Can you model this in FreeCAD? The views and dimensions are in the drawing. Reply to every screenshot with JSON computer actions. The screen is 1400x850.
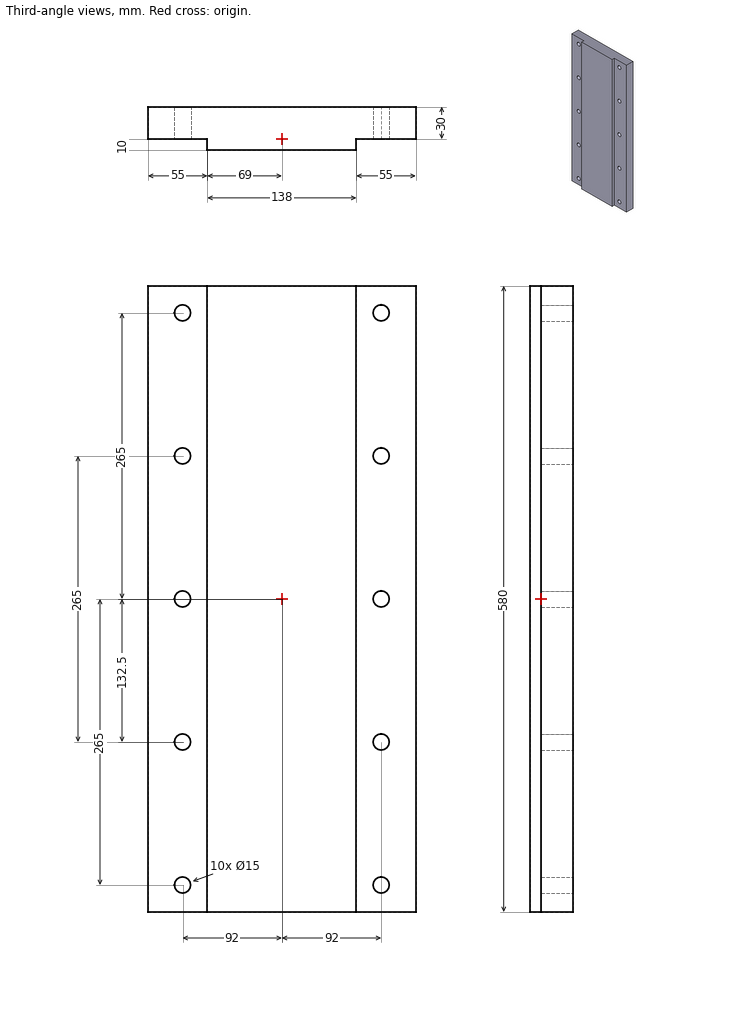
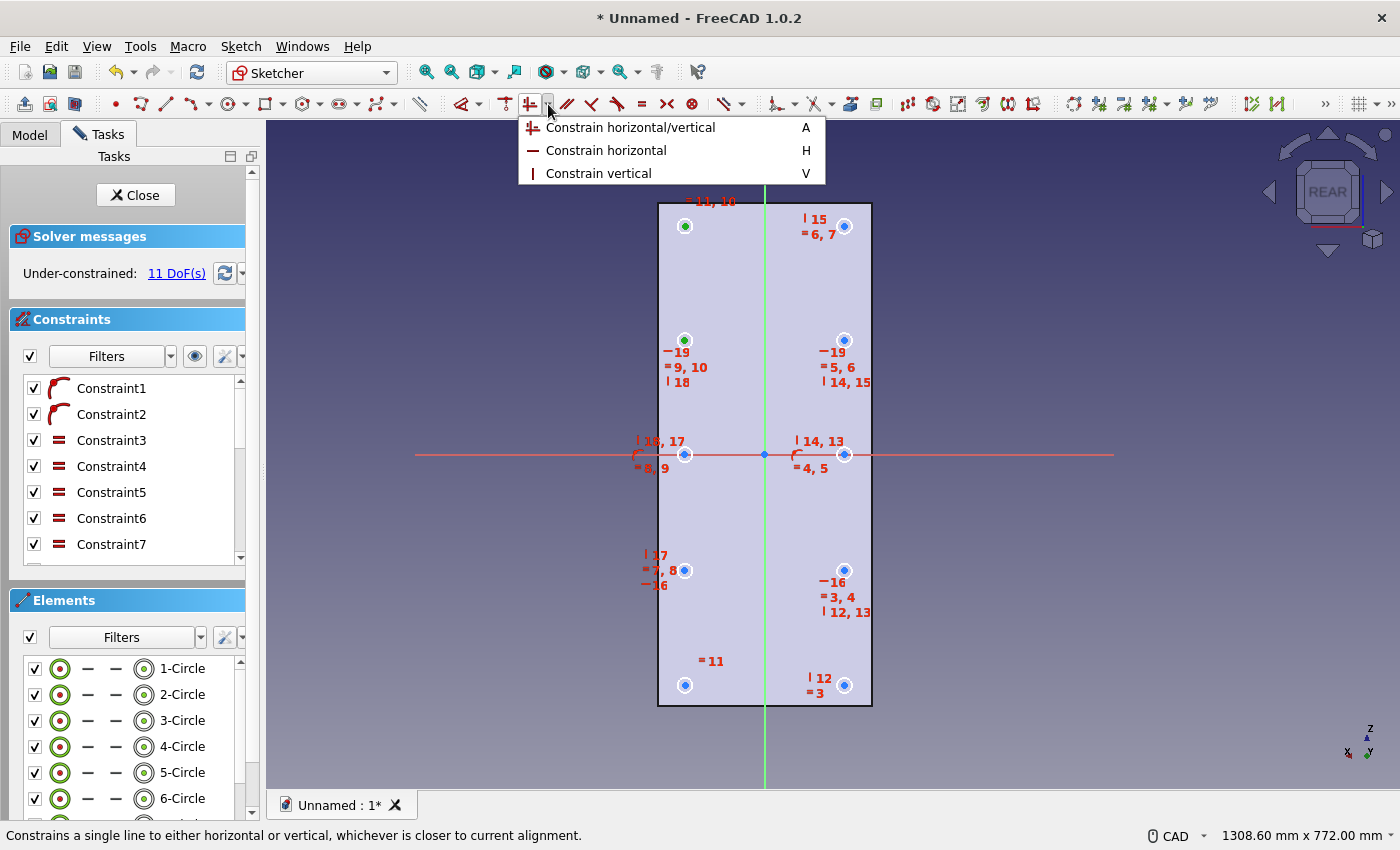
{"action": "left_click", "coordinate": [672, 174]}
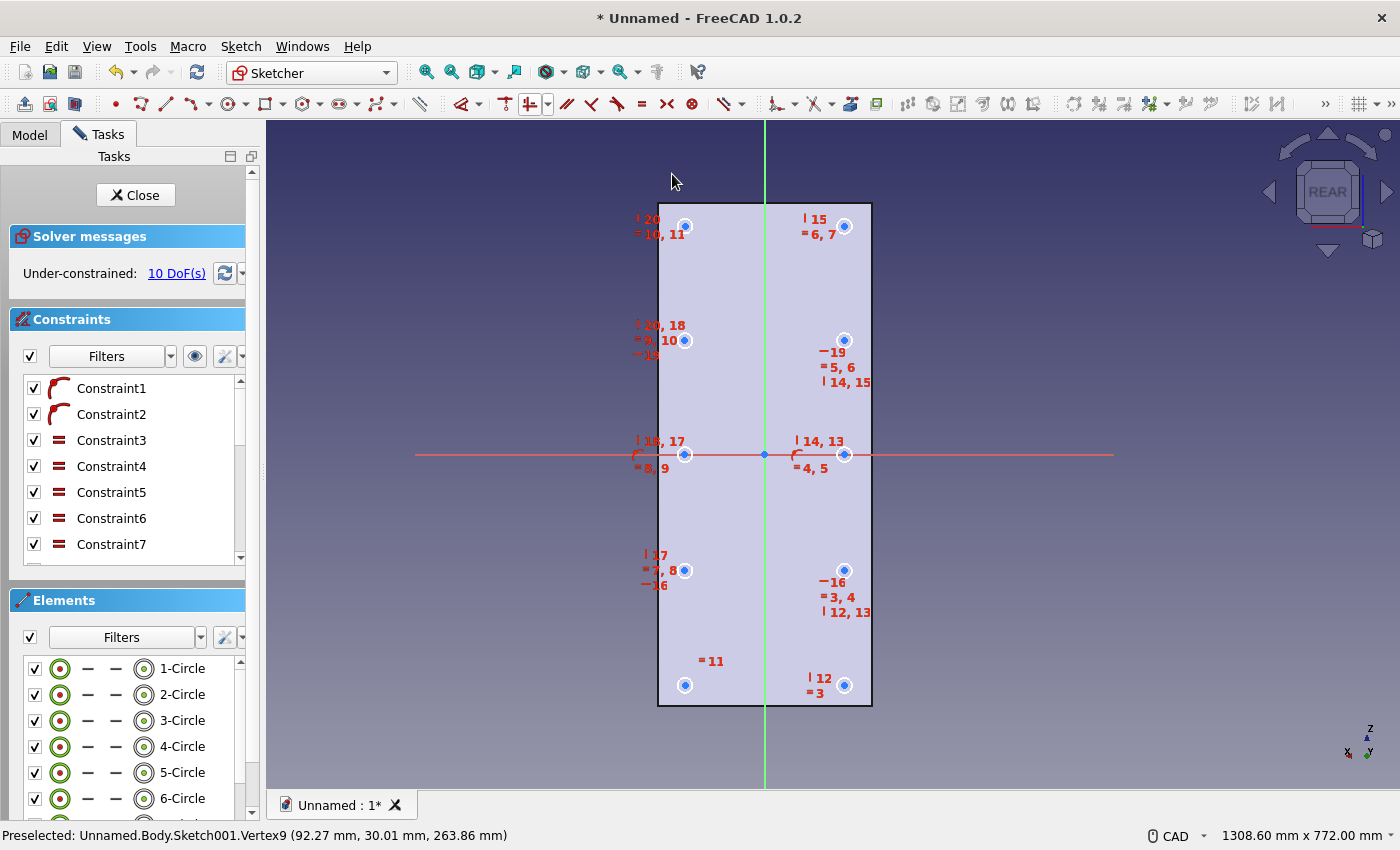
{"action": "left_click", "coordinate": [844, 226]}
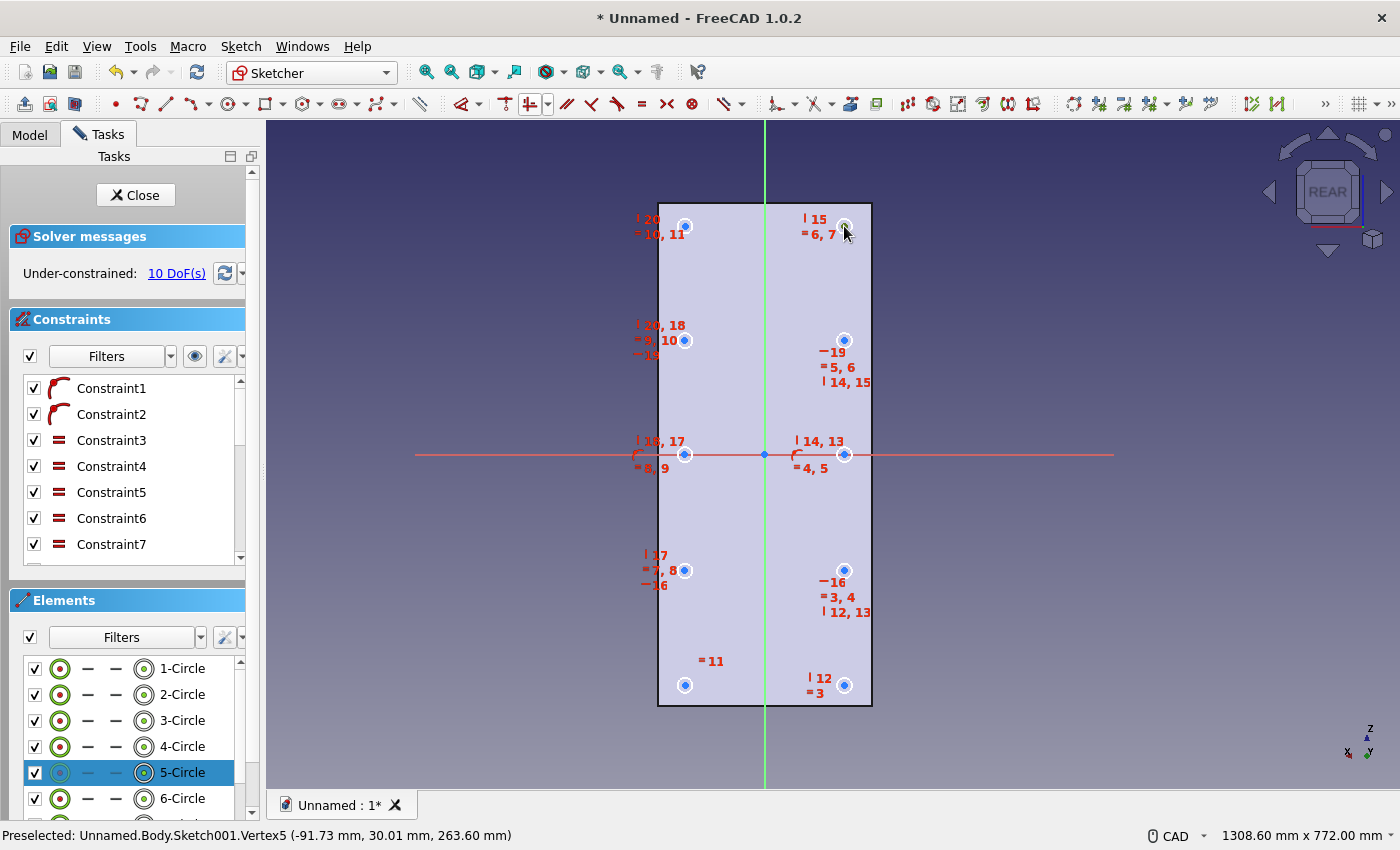
{"action": "left_click", "coordinate": [685, 226]}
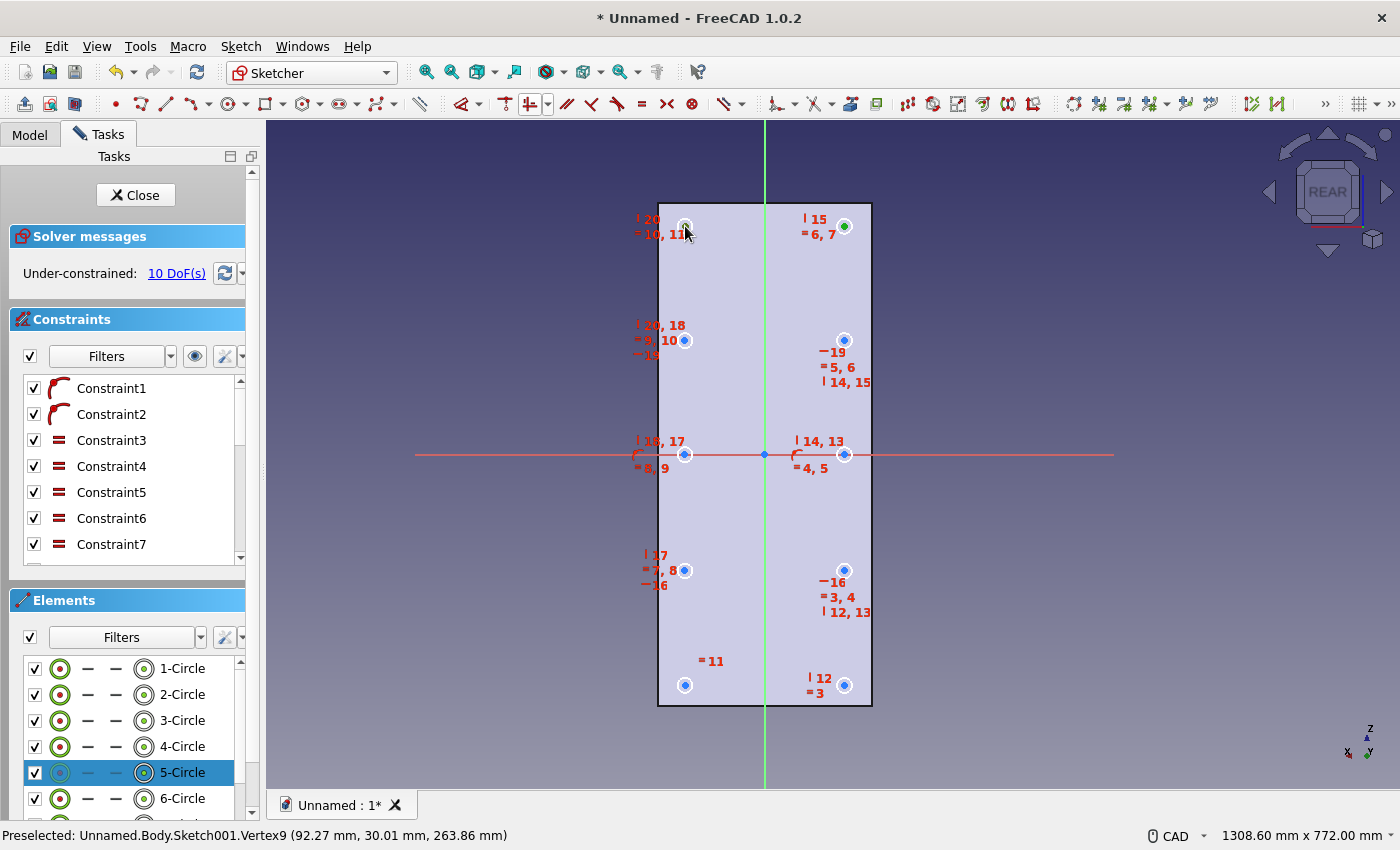
{"action": "key", "text": "h"}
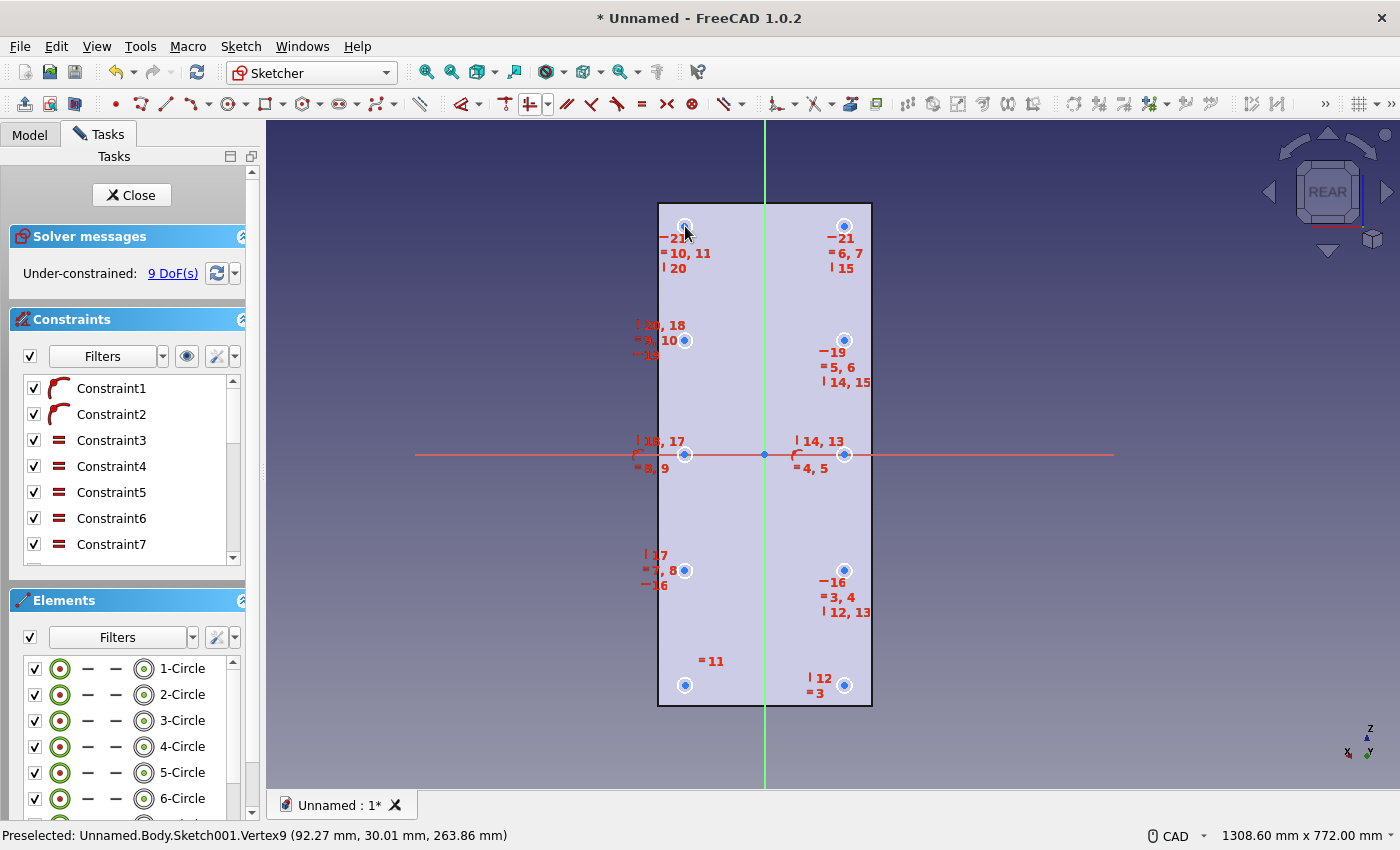
{"action": "left_click", "coordinate": [685, 571]}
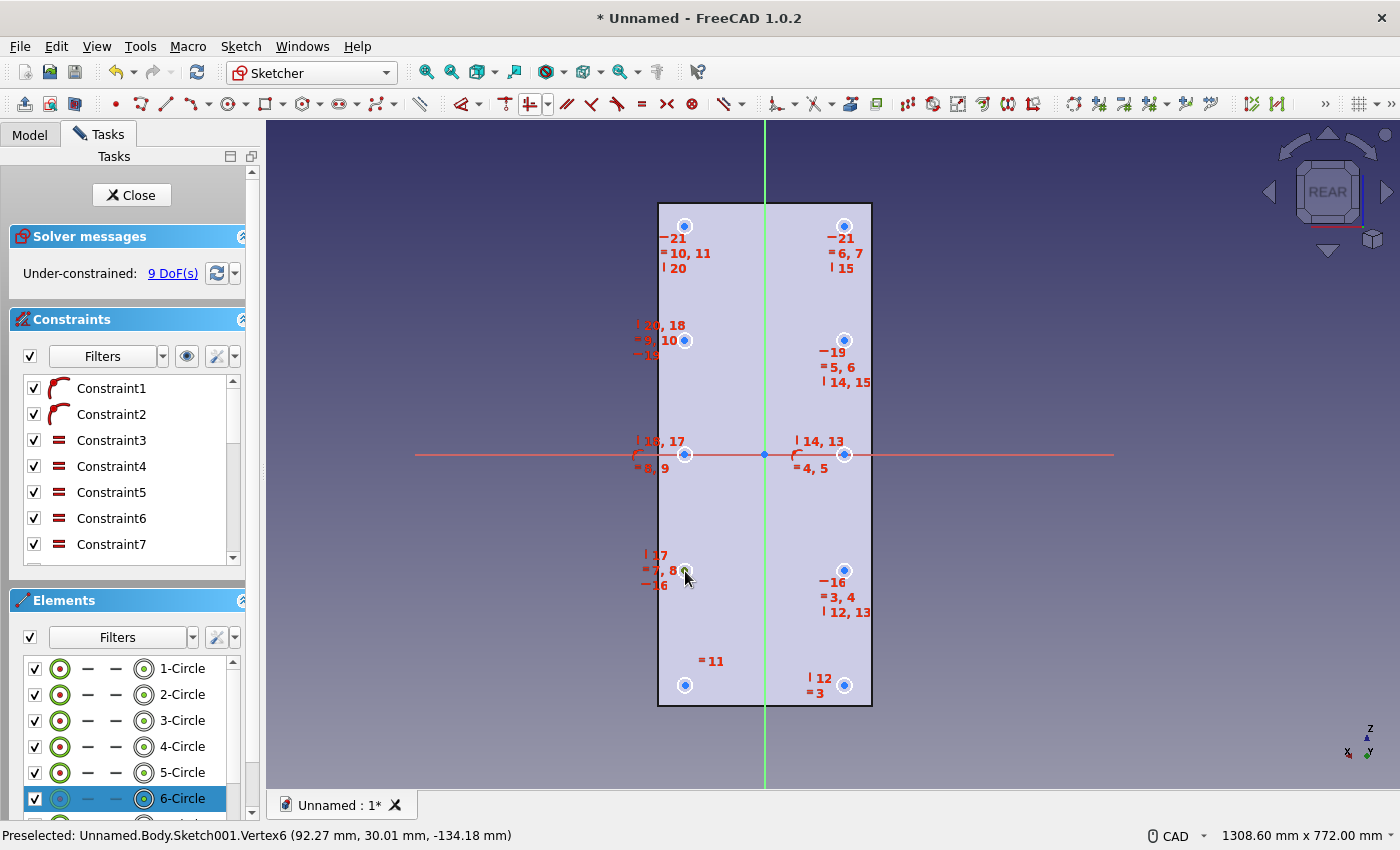
{"action": "left_click", "coordinate": [685, 685]}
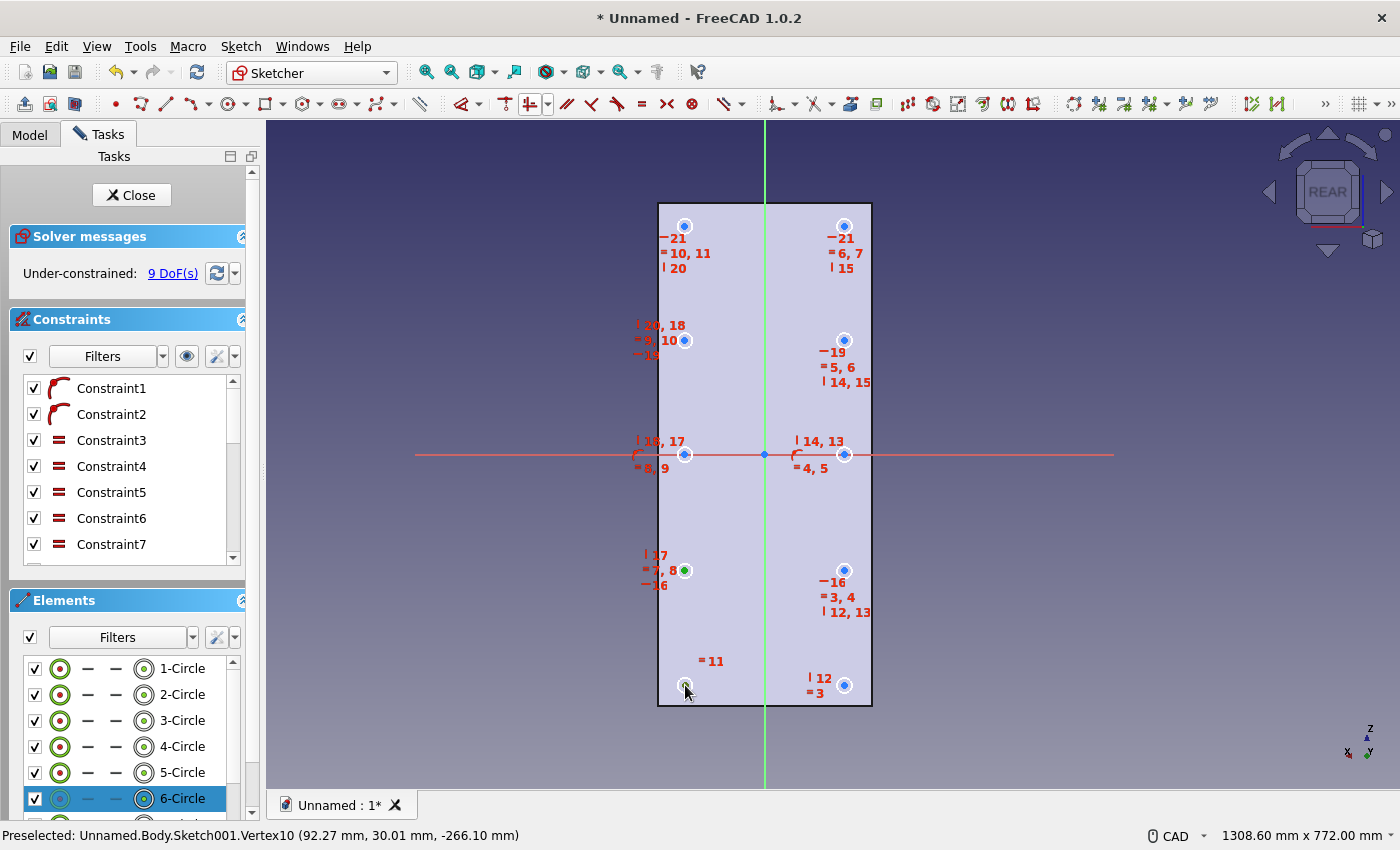
{"action": "key", "text": "v"}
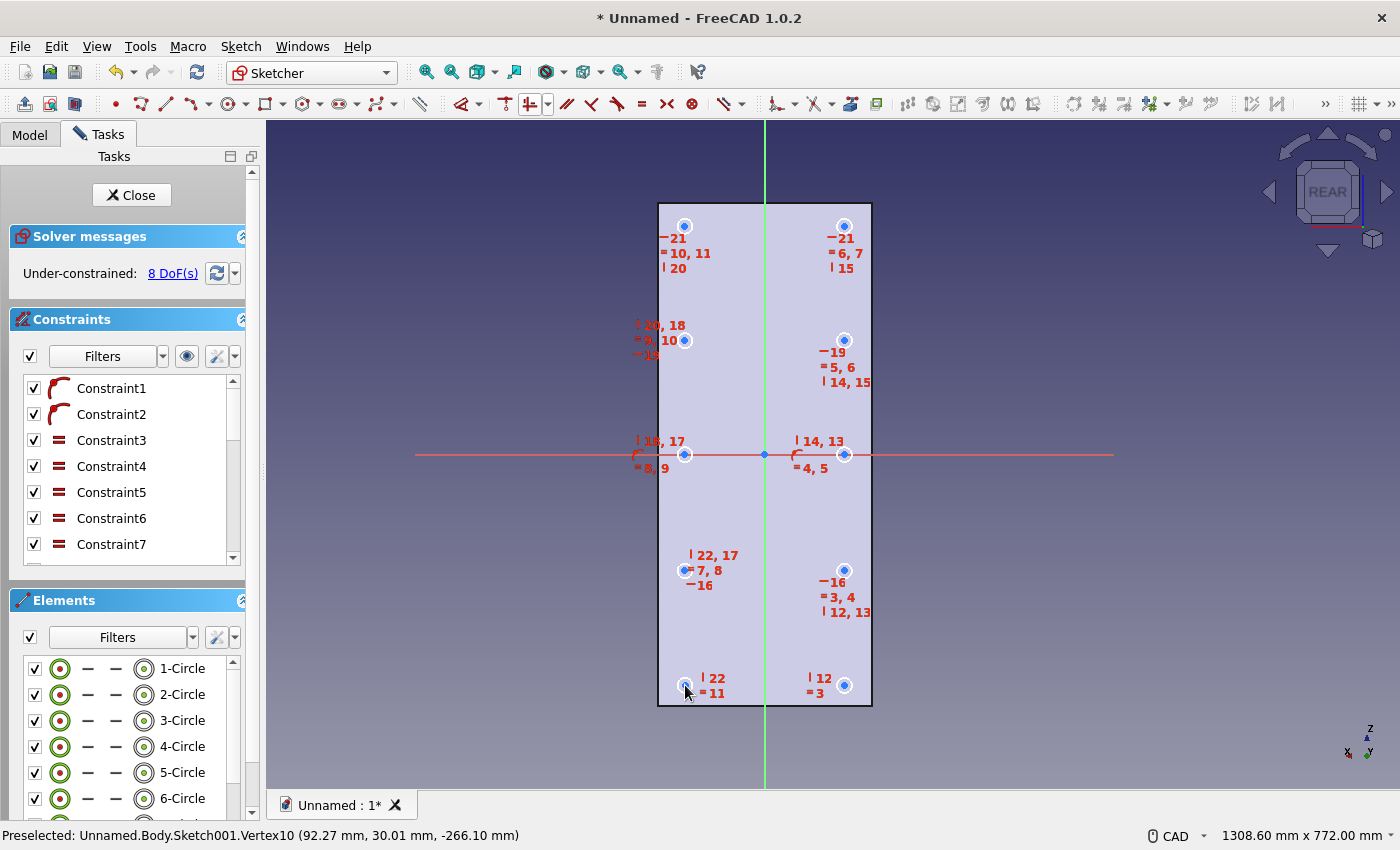
{"action": "left_click", "coordinate": [844, 685]}